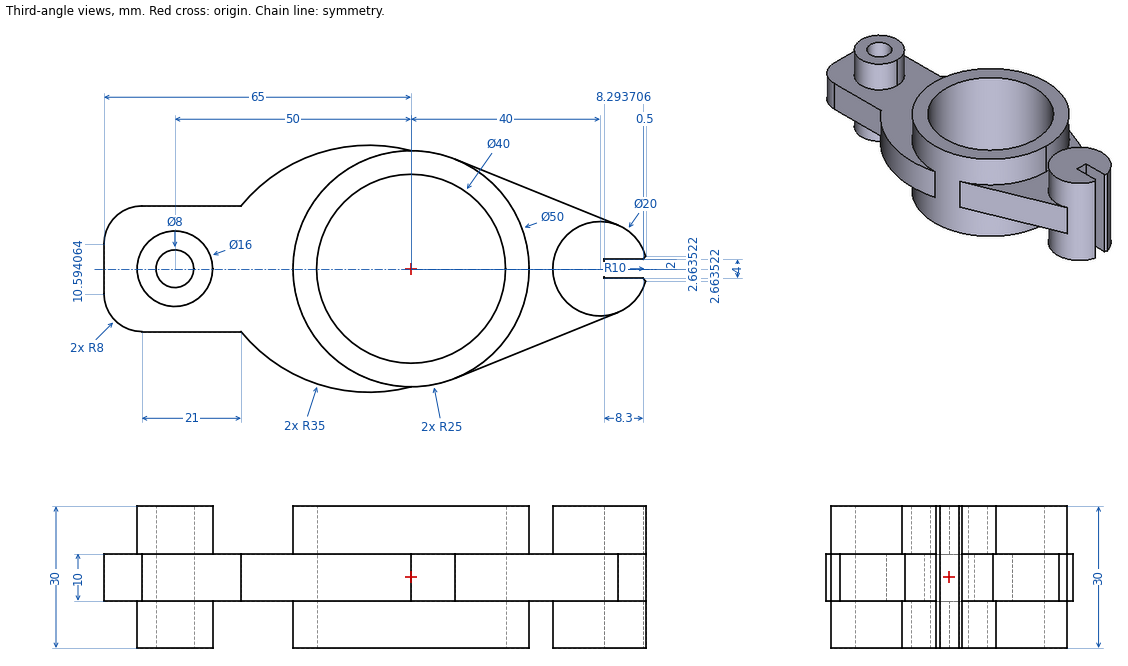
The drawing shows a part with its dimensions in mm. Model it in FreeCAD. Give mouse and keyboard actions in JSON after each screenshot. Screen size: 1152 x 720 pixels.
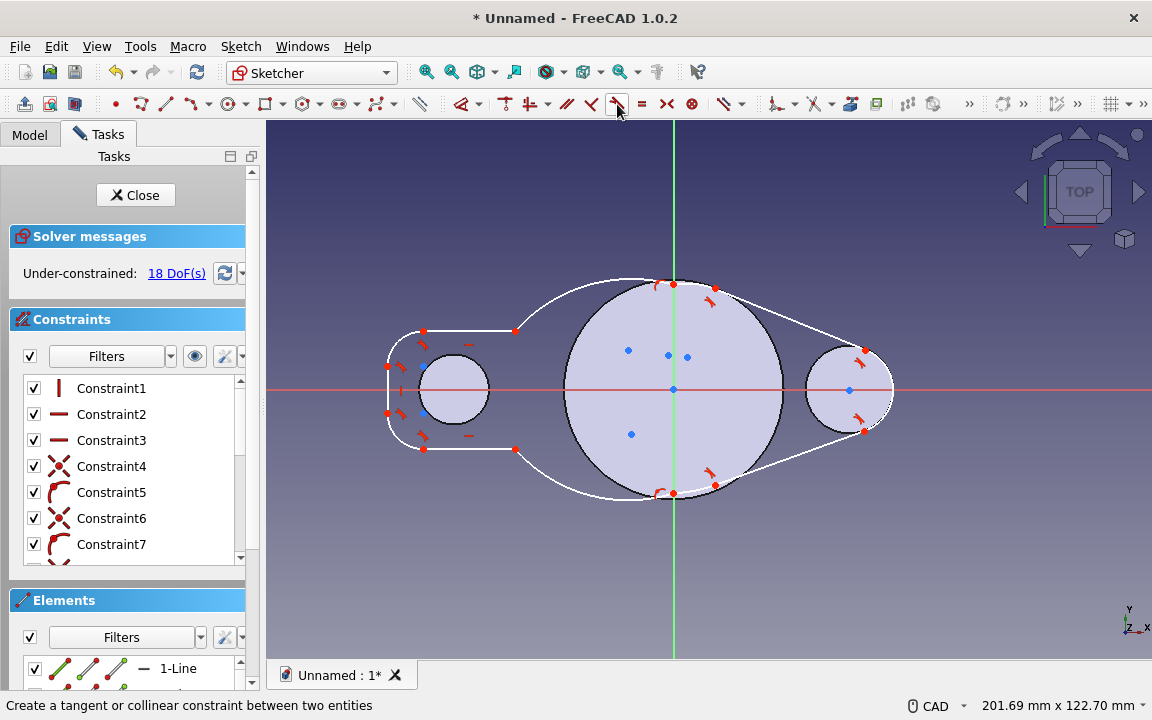
{"action": "left_click", "coordinate": [686, 492]}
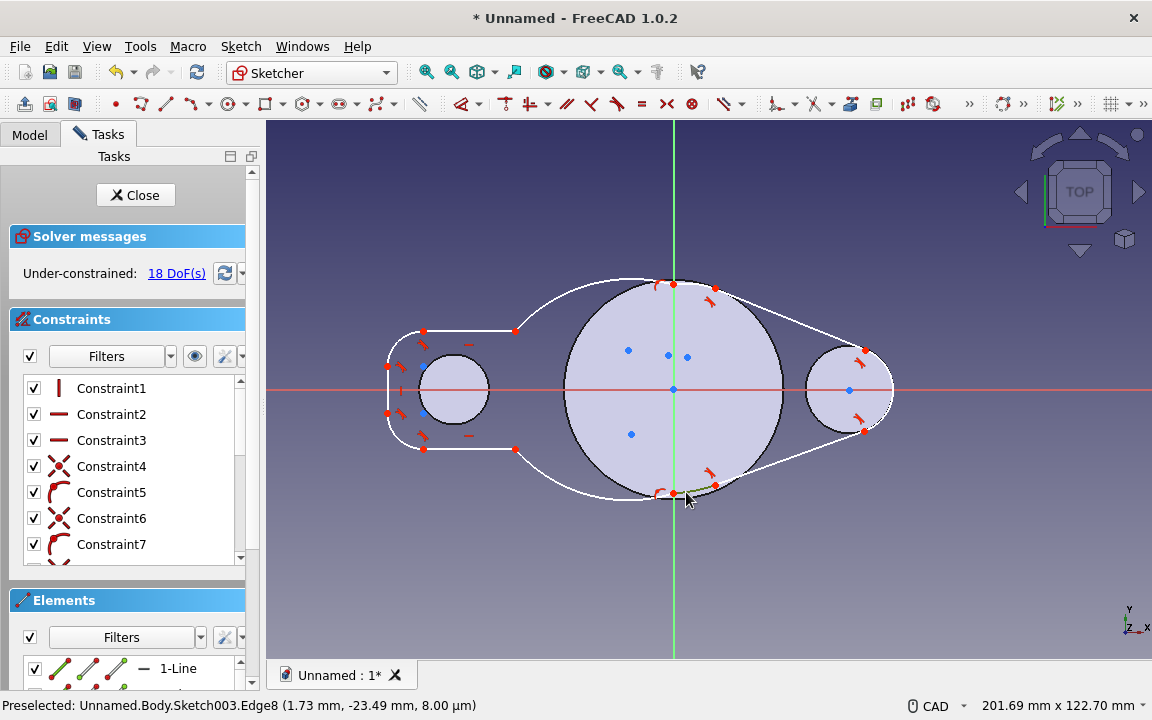
{"action": "left_click", "coordinate": [703, 285]}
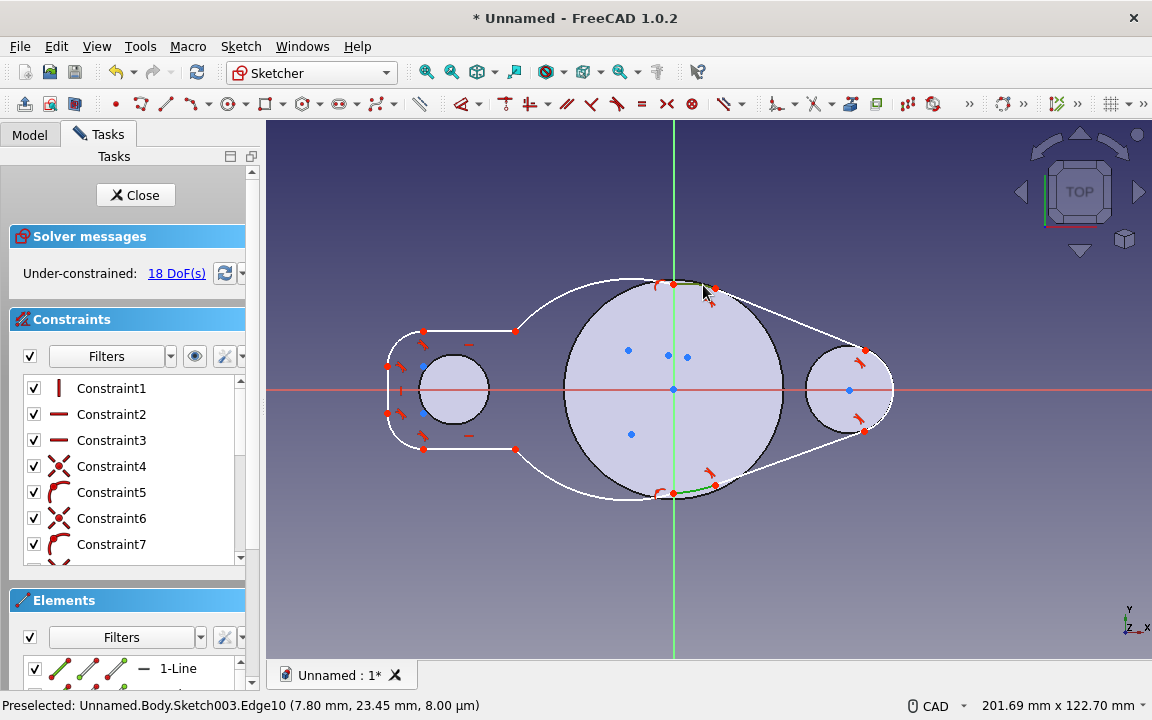
{"action": "left_click", "coordinate": [505, 104]}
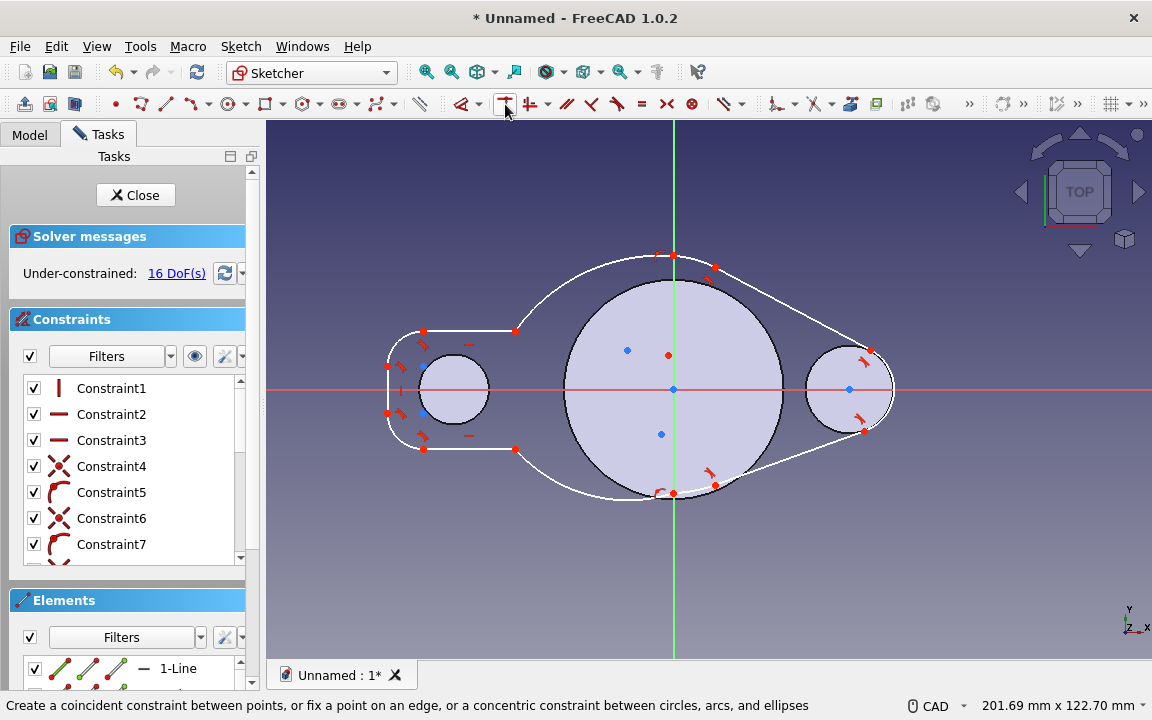
{"action": "left_click_drag", "start_coordinate": [658, 345], "coordinate": [684, 400]}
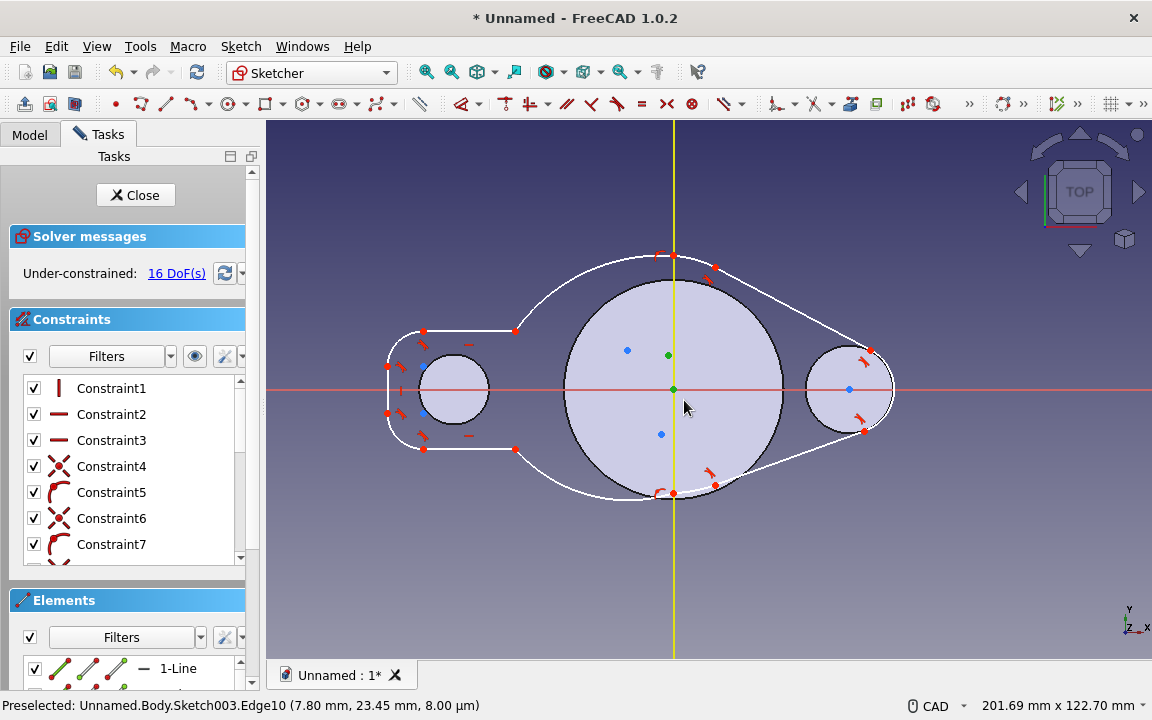
{"action": "left_click", "coordinate": [505, 104]}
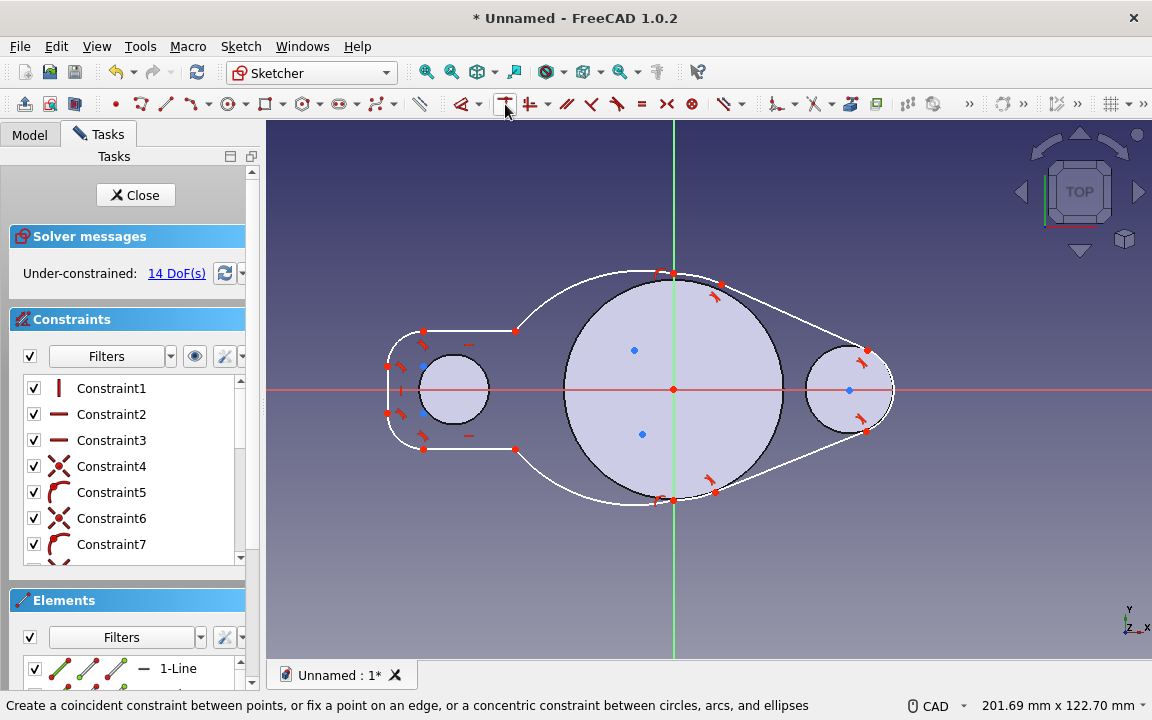
{"action": "left_click", "coordinate": [686, 499]}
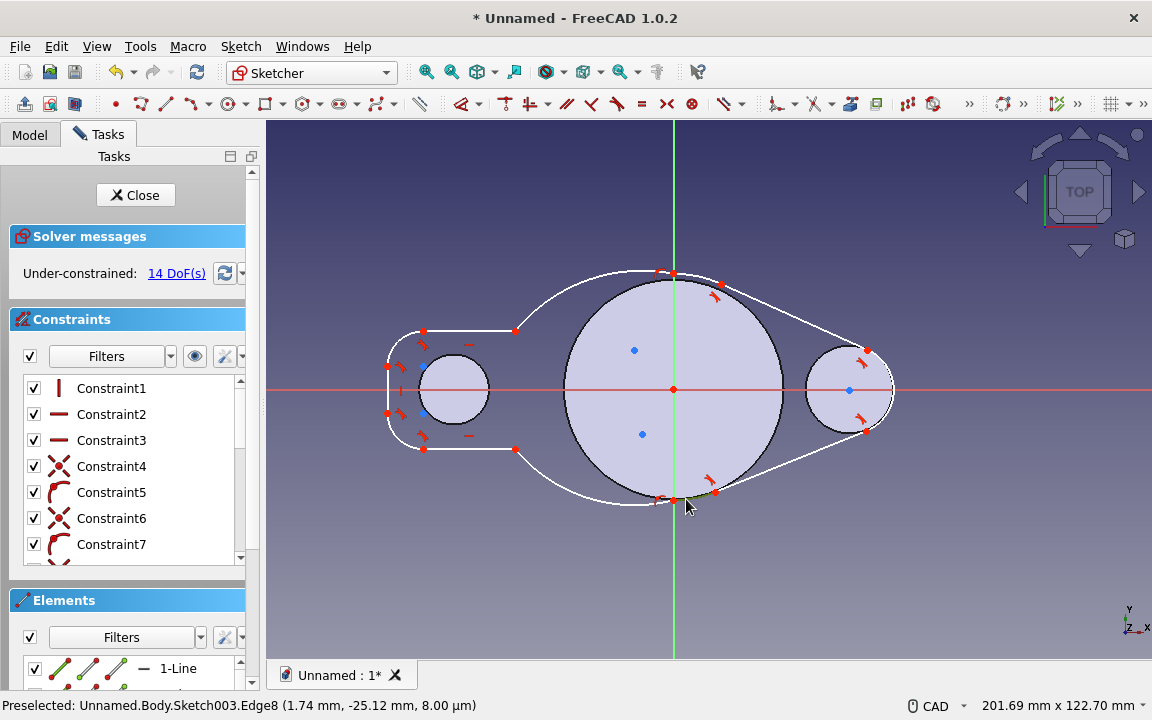
{"action": "left_click", "coordinate": [707, 279]}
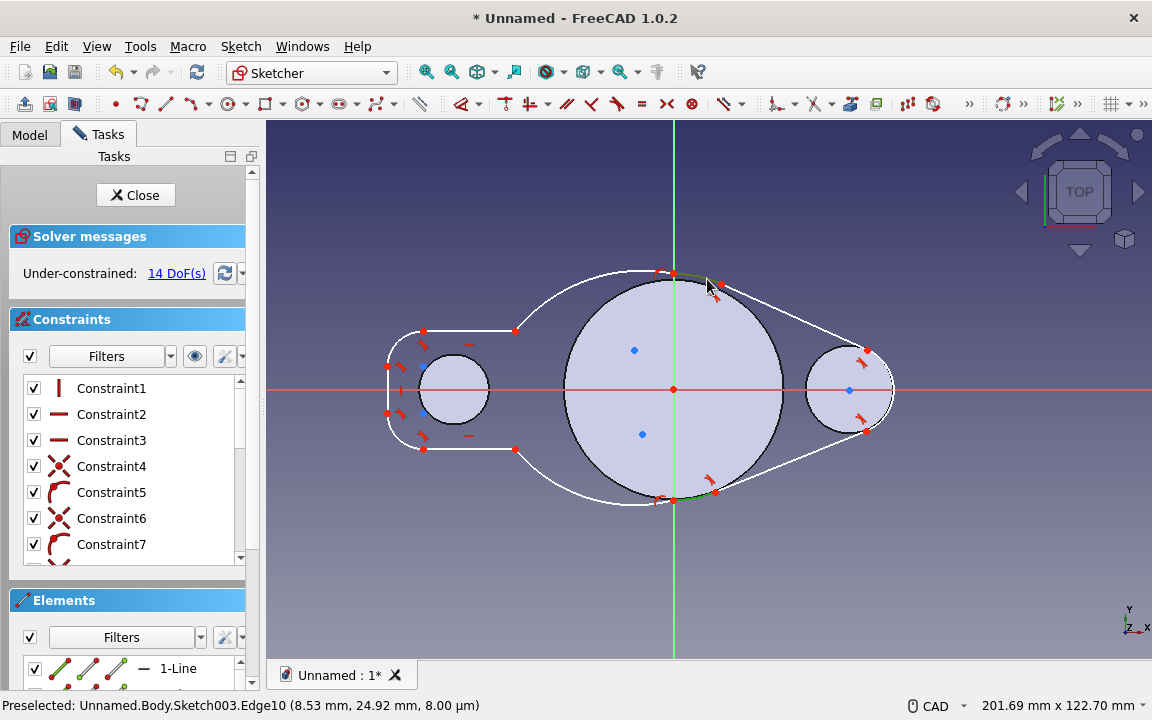
{"action": "key", "text": "e"}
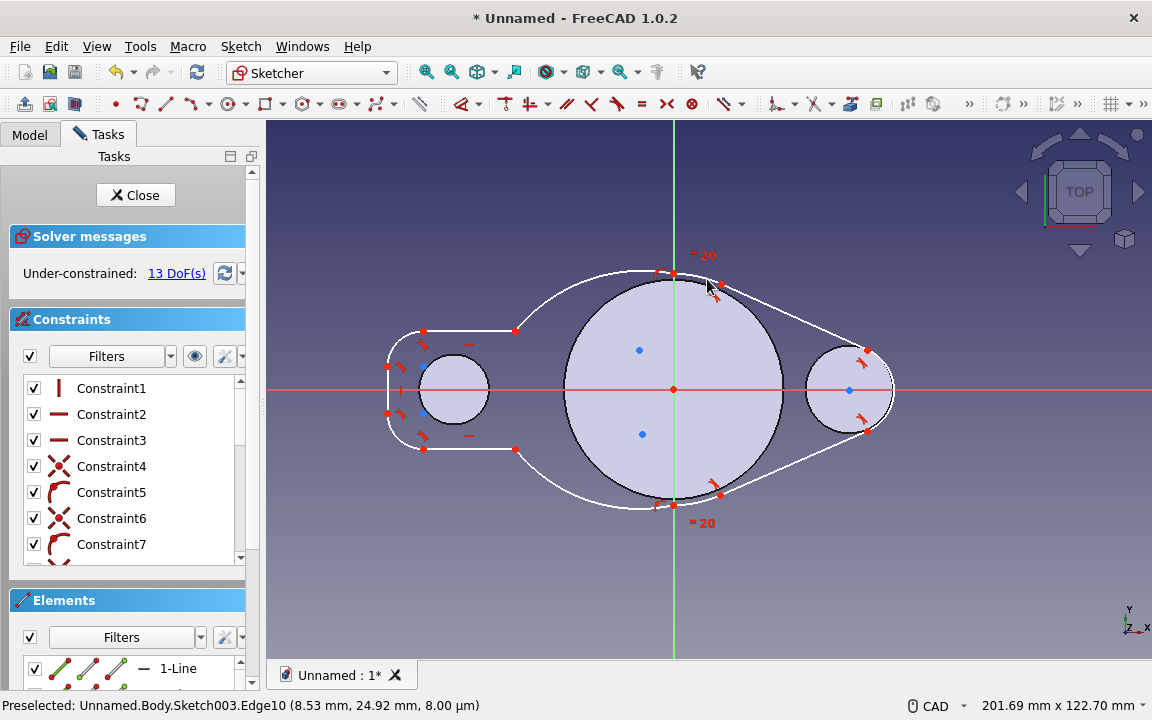
{"action": "left_click", "coordinate": [555, 484]}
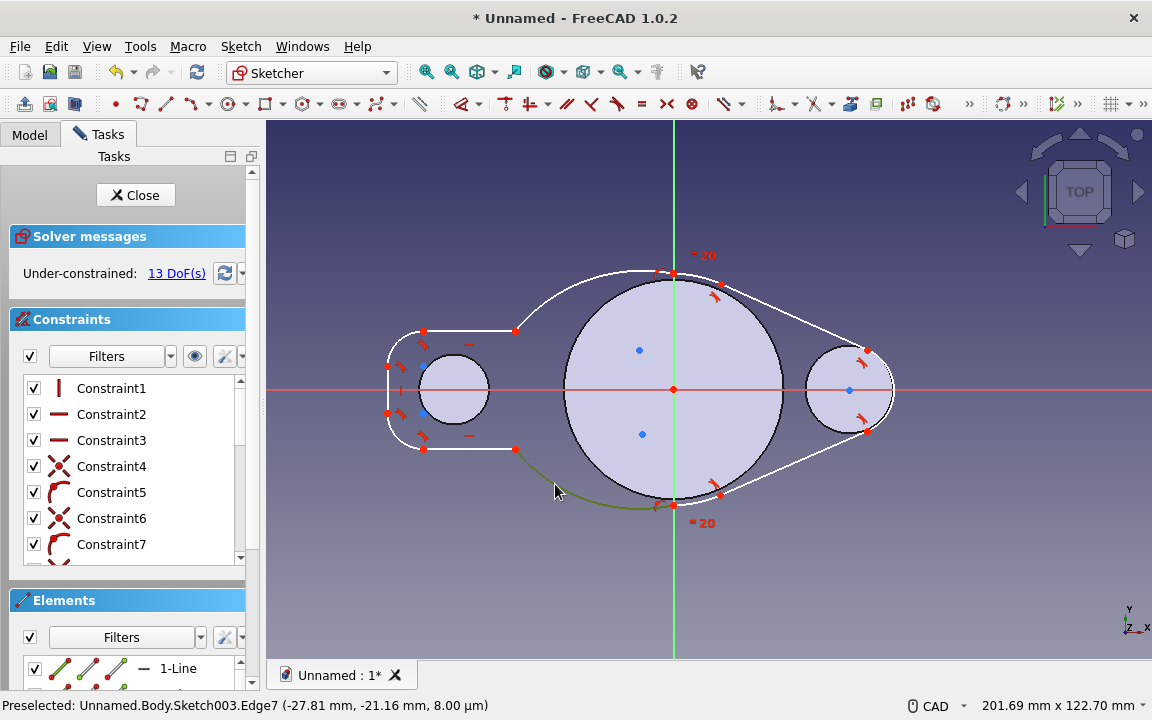
{"action": "left_click", "coordinate": [621, 272]}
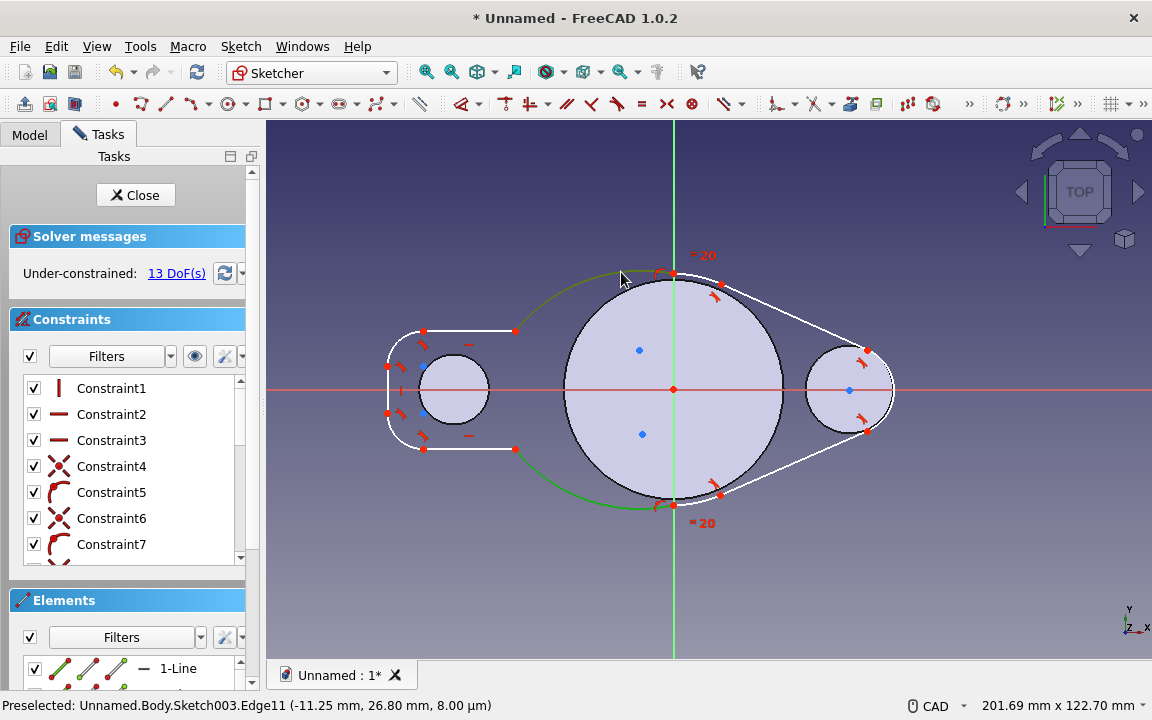
{"action": "left_click", "coordinate": [642, 104]}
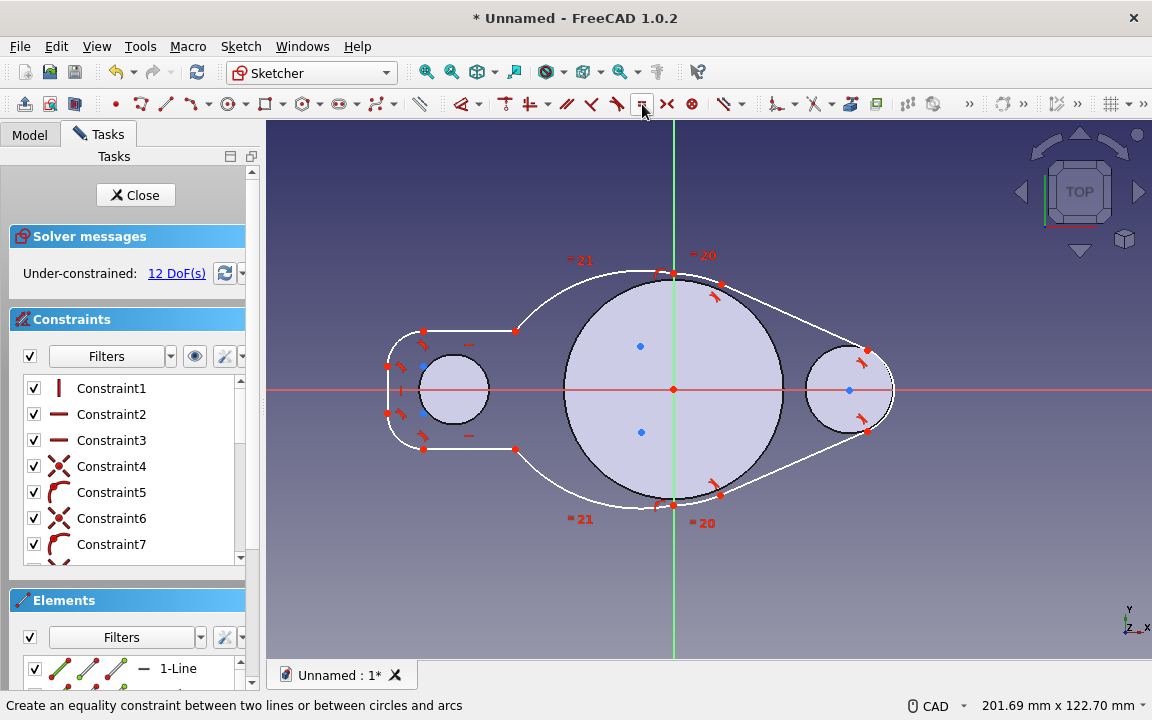
{"action": "left_click", "coordinate": [391, 430]}